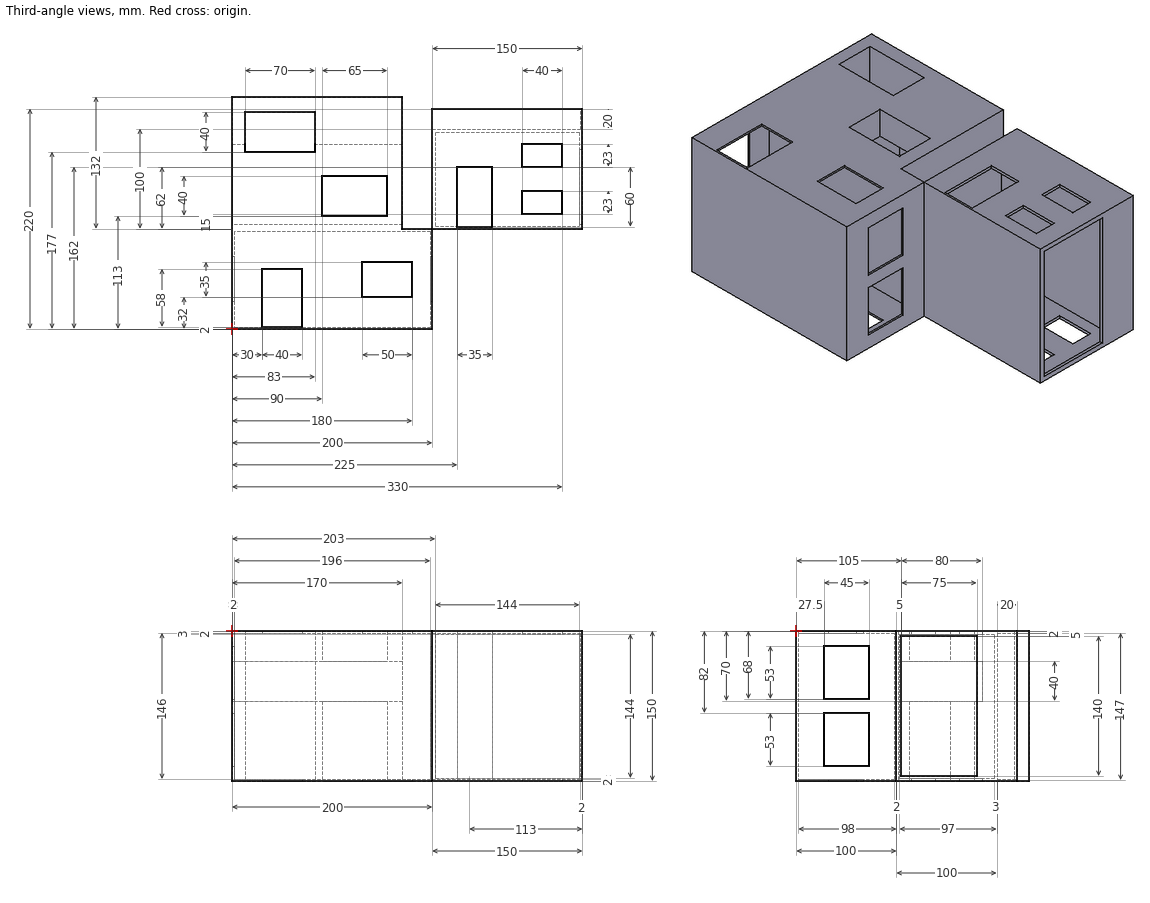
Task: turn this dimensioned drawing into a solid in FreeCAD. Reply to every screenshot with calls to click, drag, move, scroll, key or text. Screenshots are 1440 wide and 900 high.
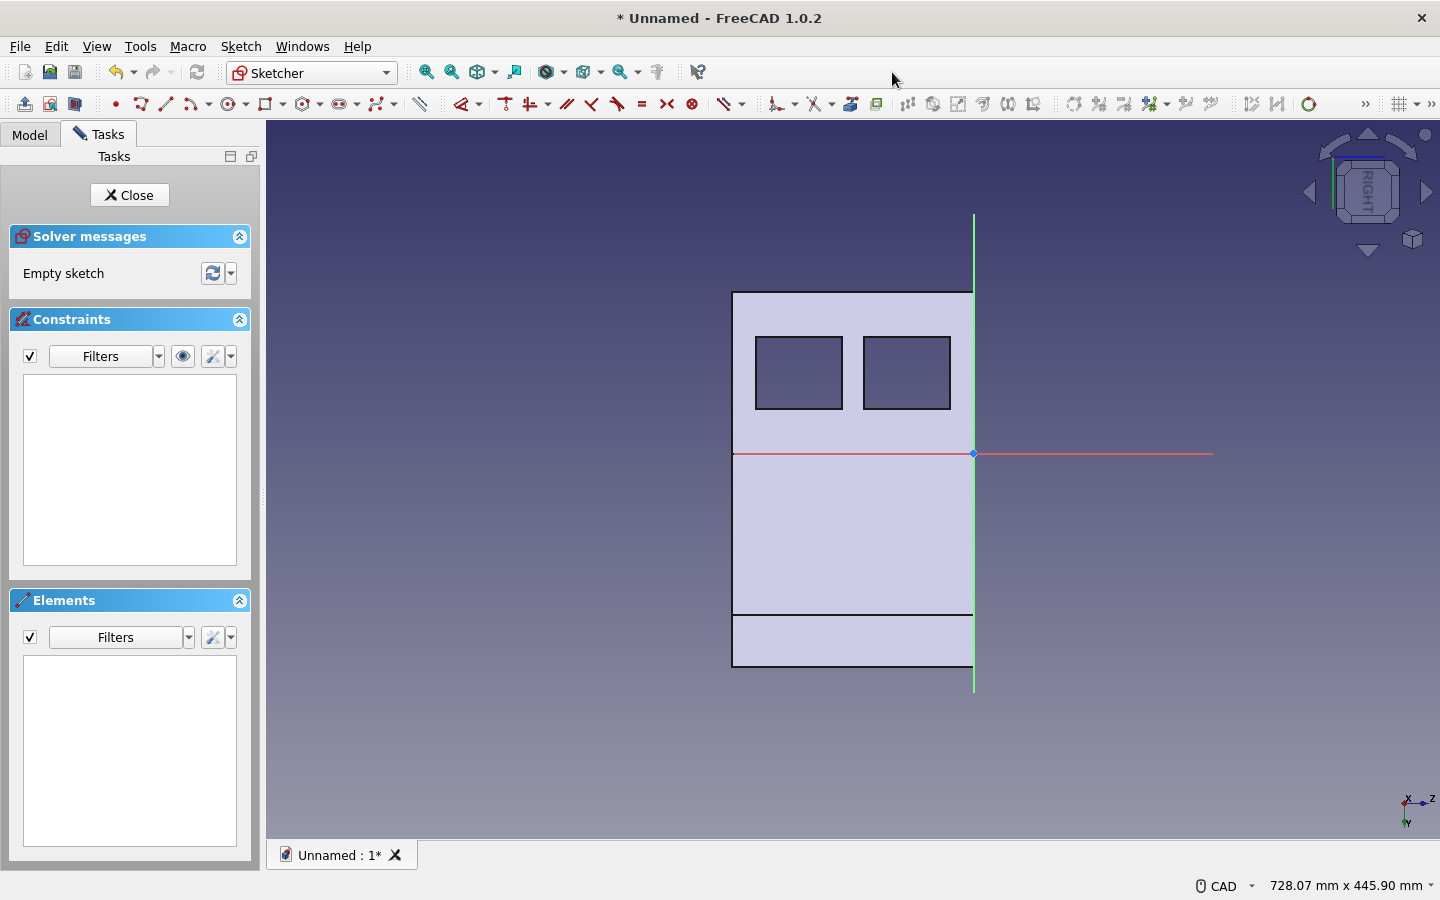
scroll(899, 541, up, 5)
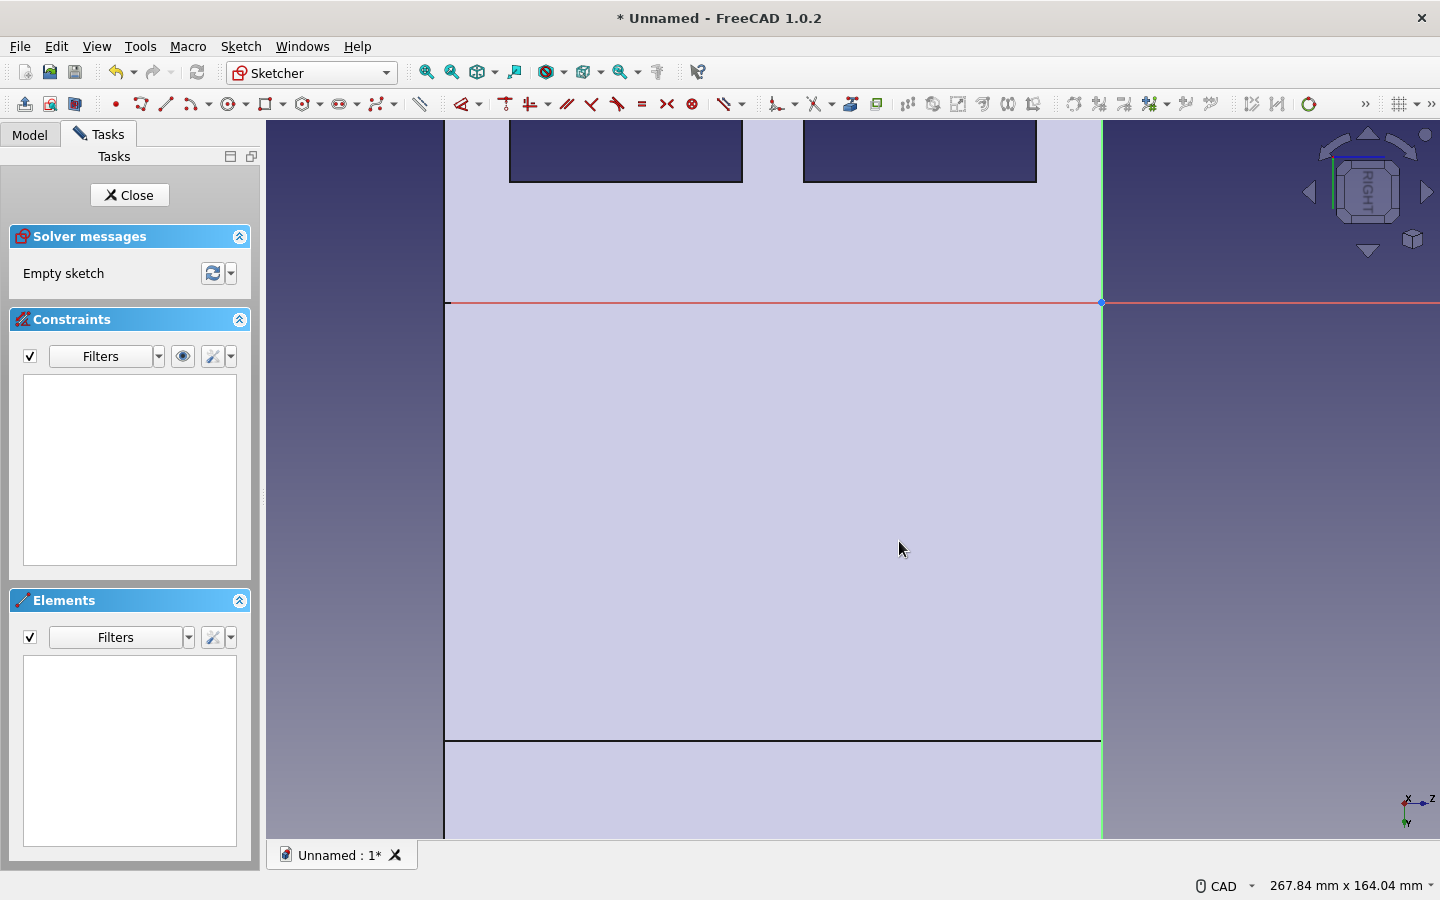
click(264, 104)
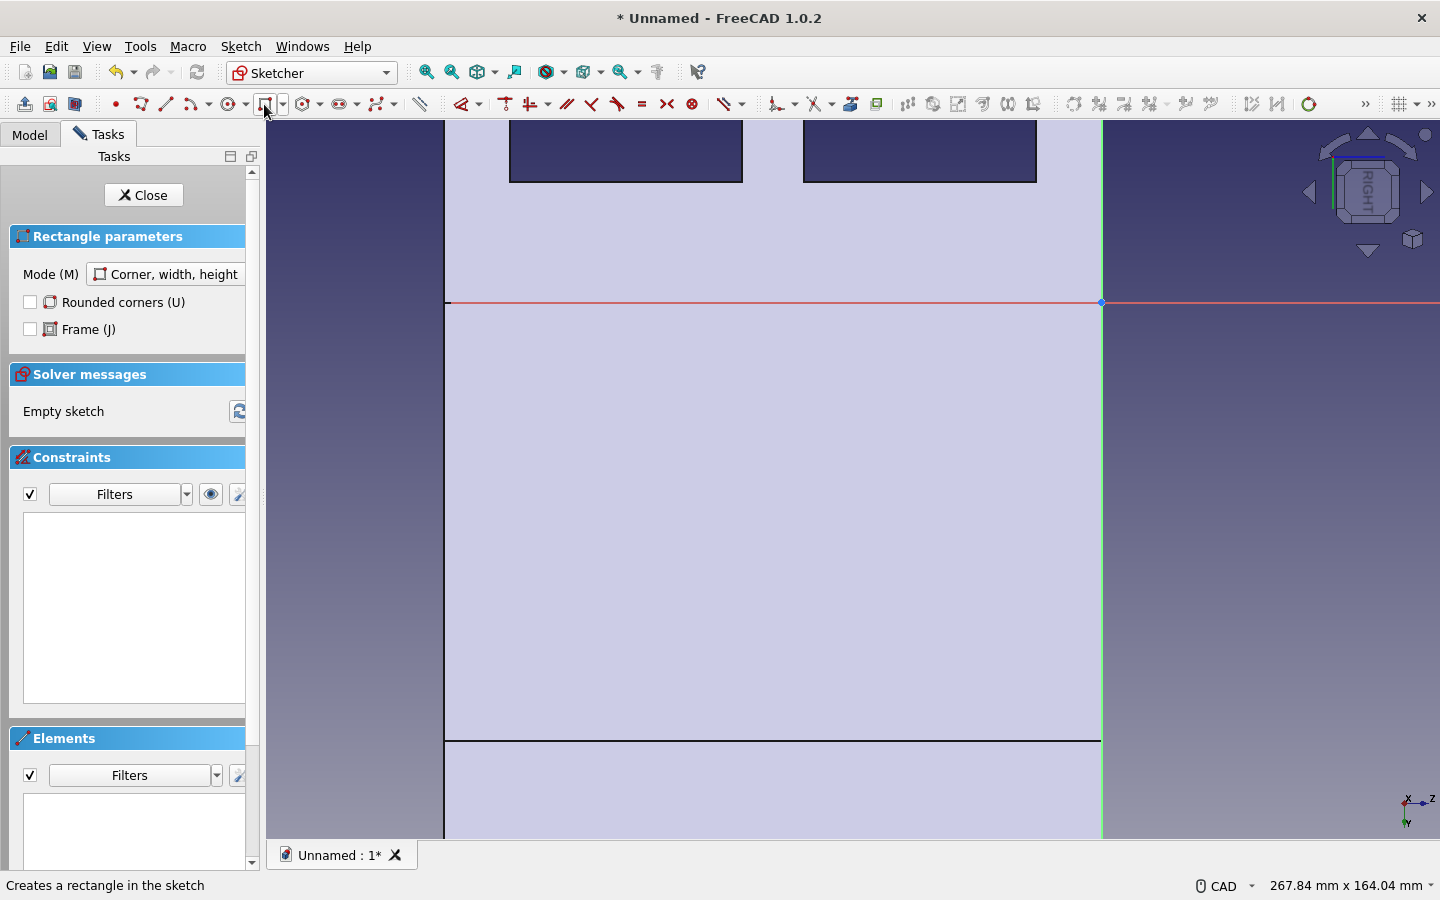
click(466, 325)
move(1080, 653)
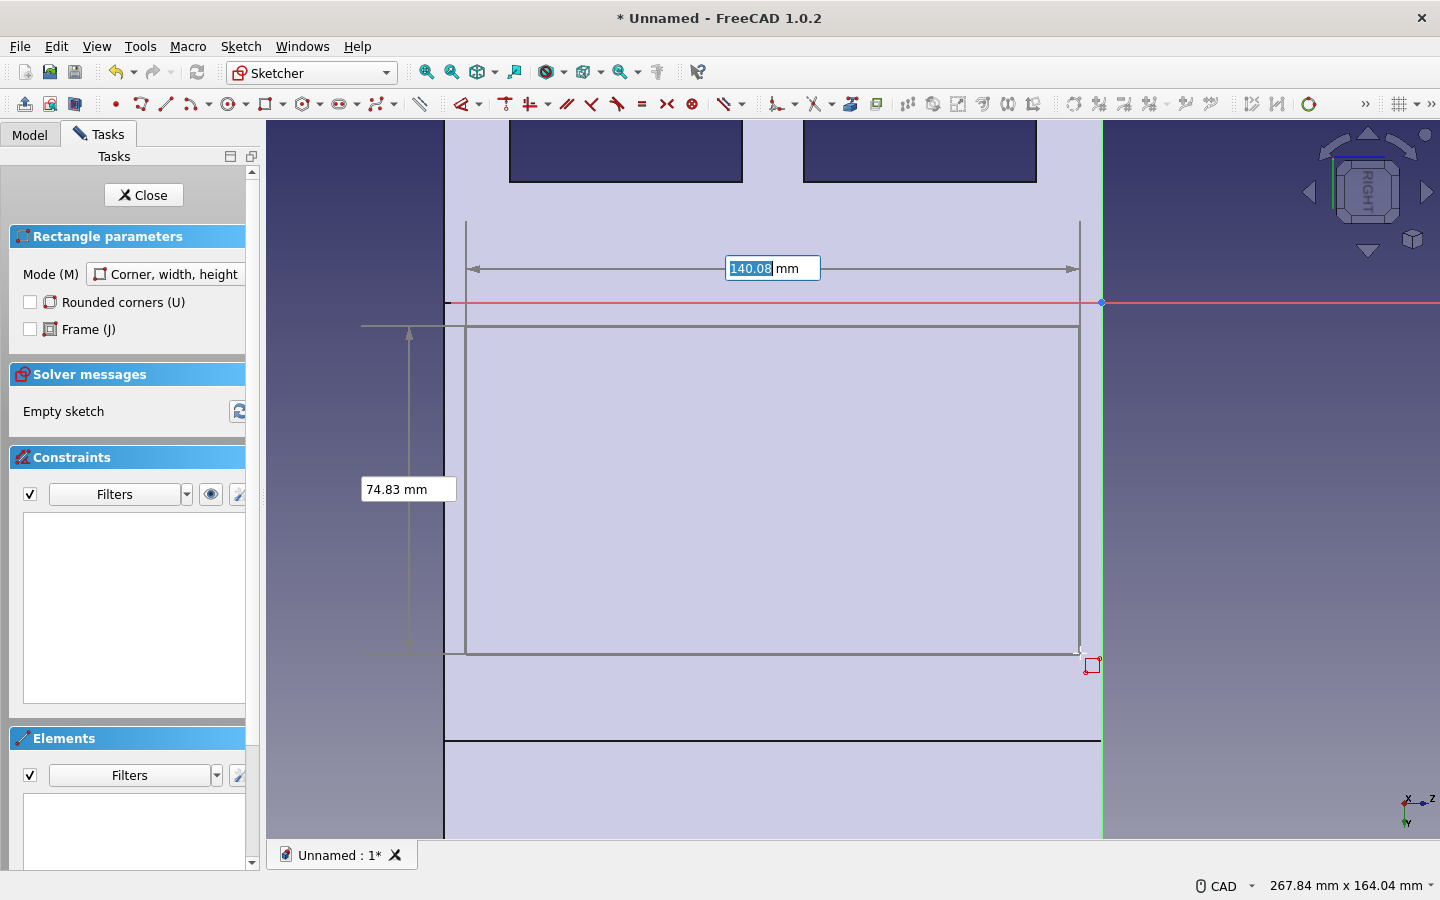
text(140)
key(Tab)
text(75)
key(Return)
key(Escape)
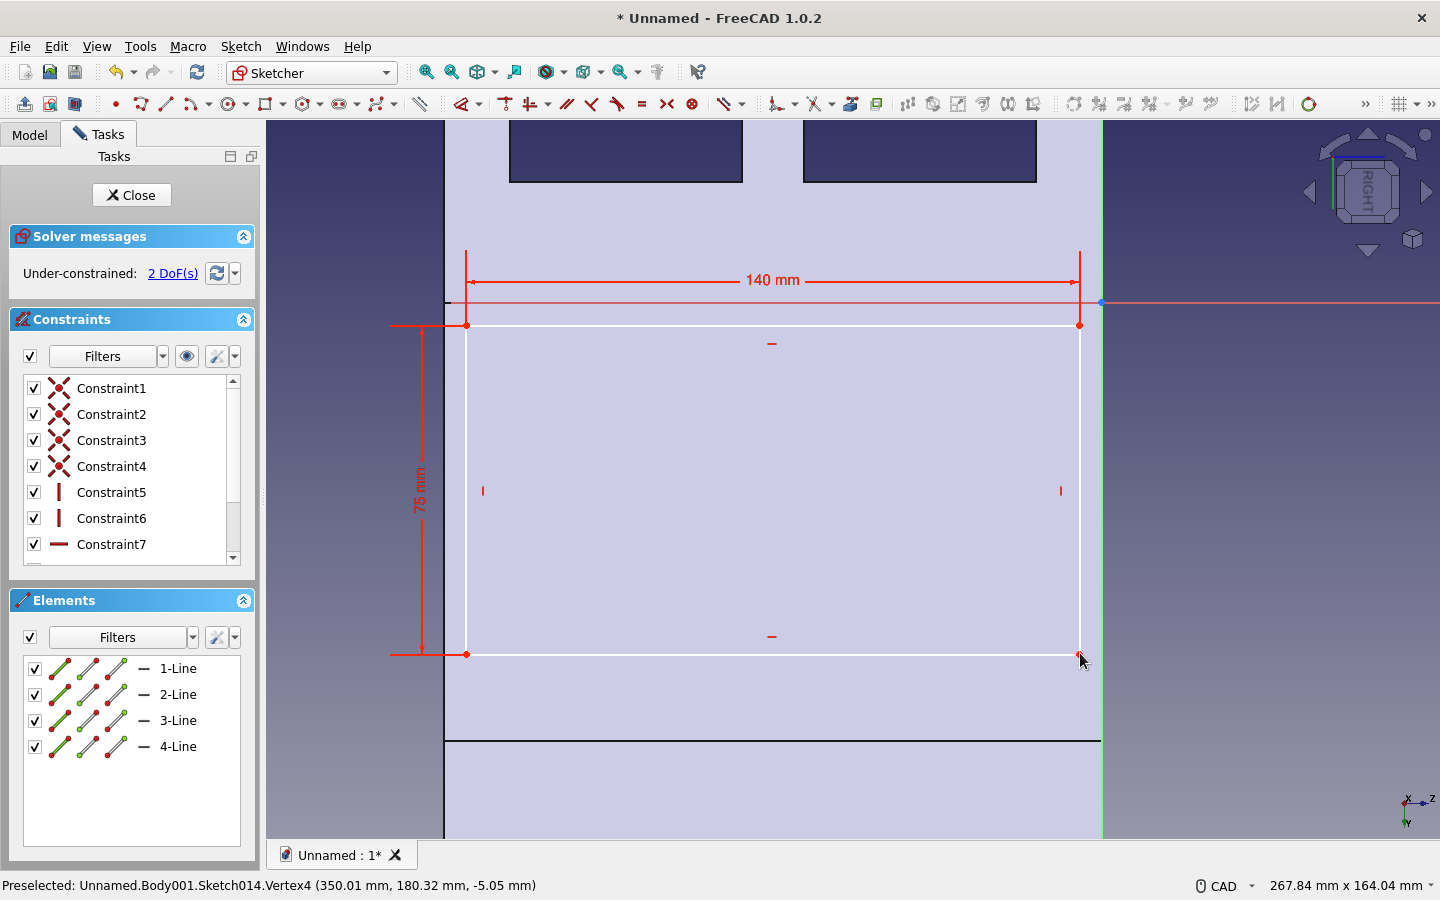
click(460, 104)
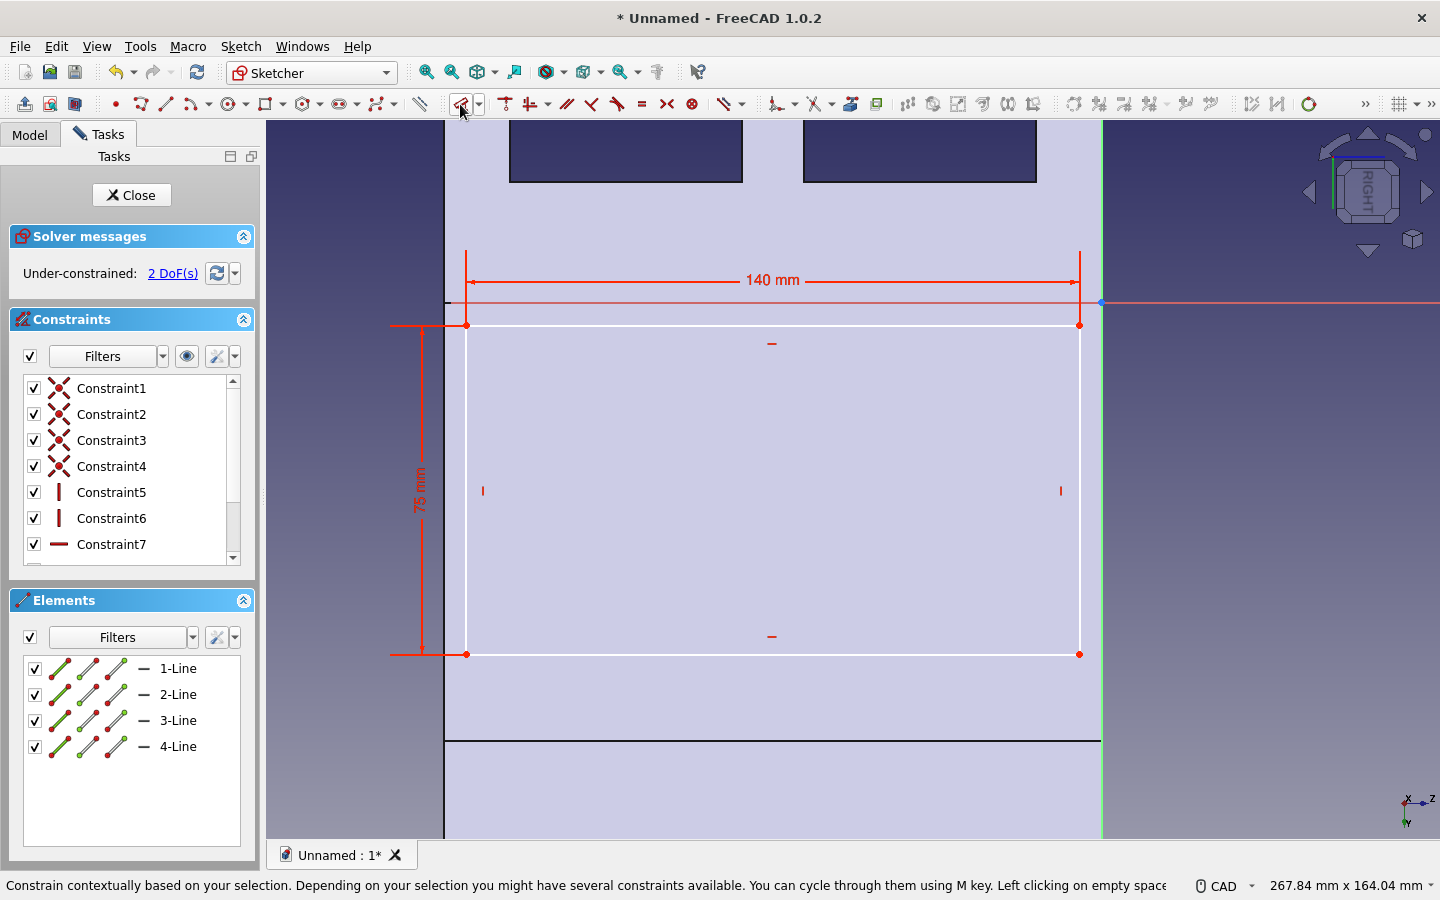
scroll(466, 326, up, 3)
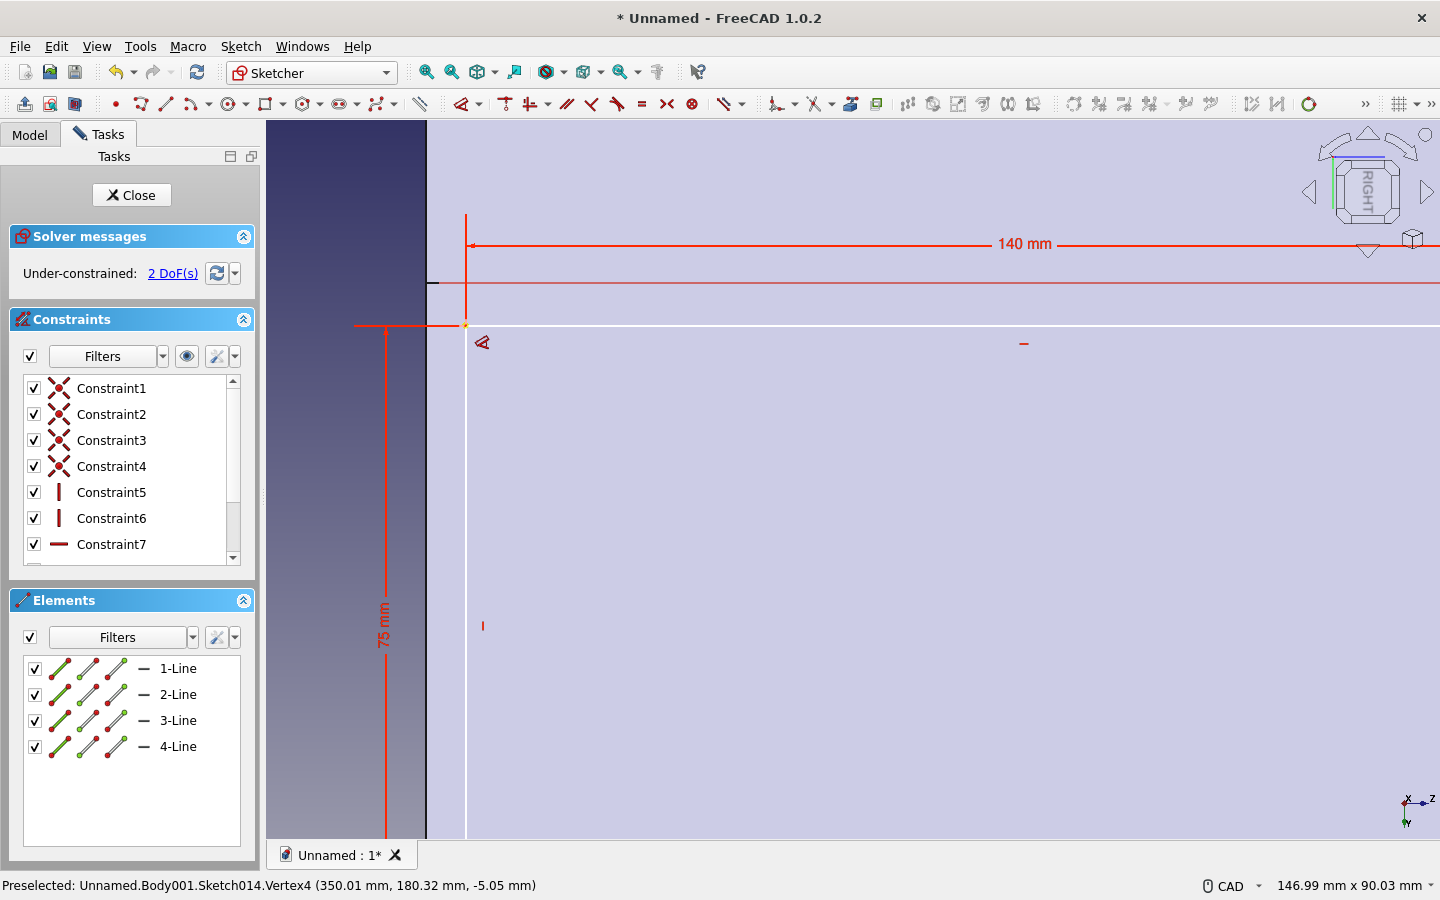
click(466, 326)
click(432, 305)